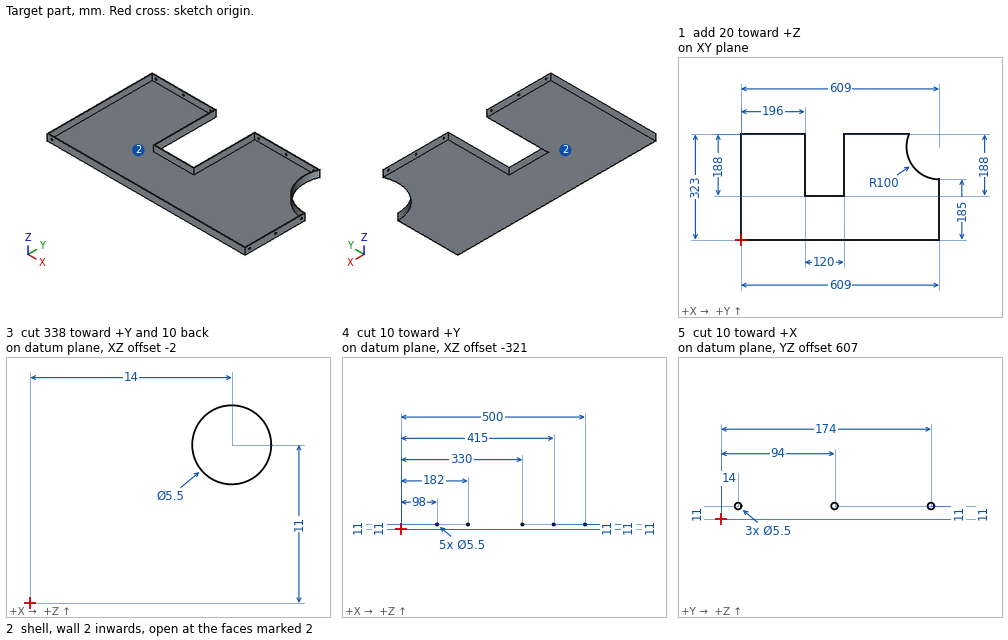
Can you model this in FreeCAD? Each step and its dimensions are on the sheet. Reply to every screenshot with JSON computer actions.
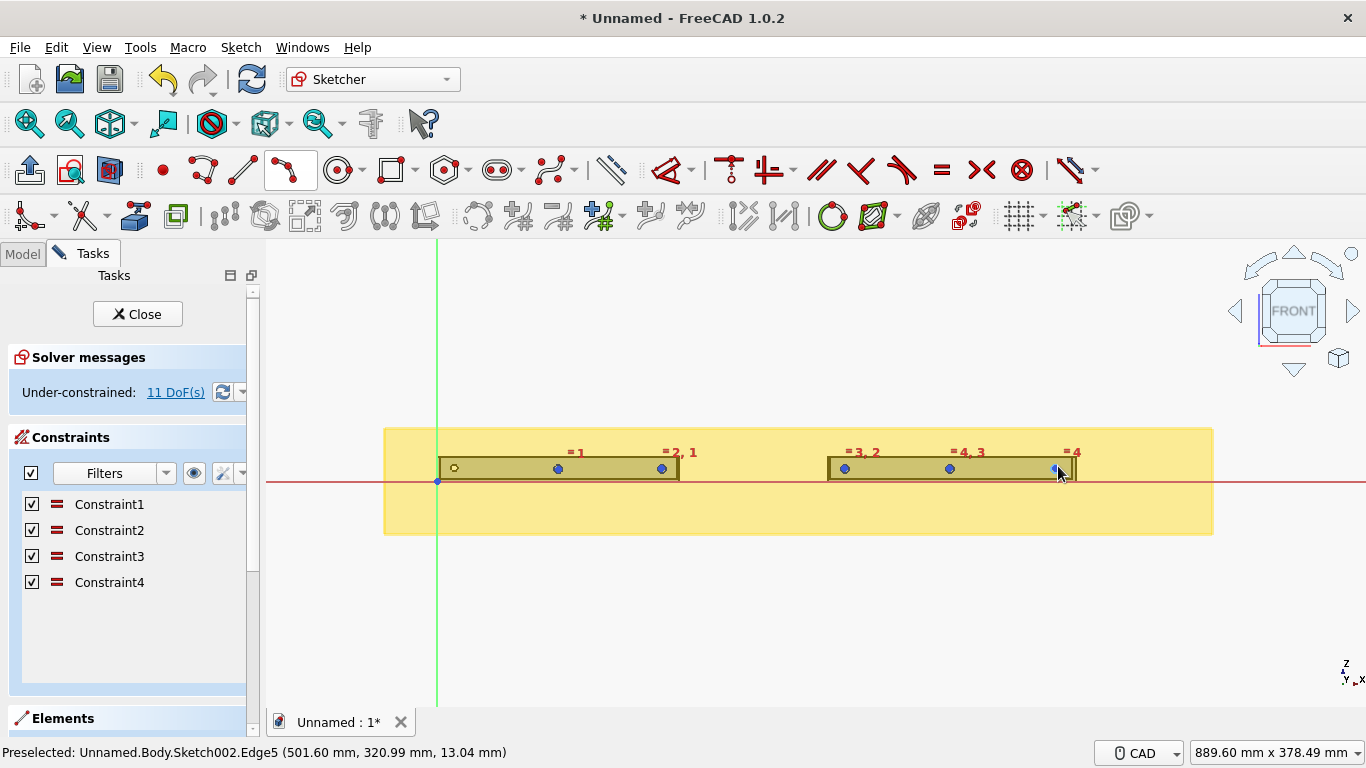
{"action": "scroll", "coordinate": [561, 466], "scroll_direction": "up", "scroll_amount": 9}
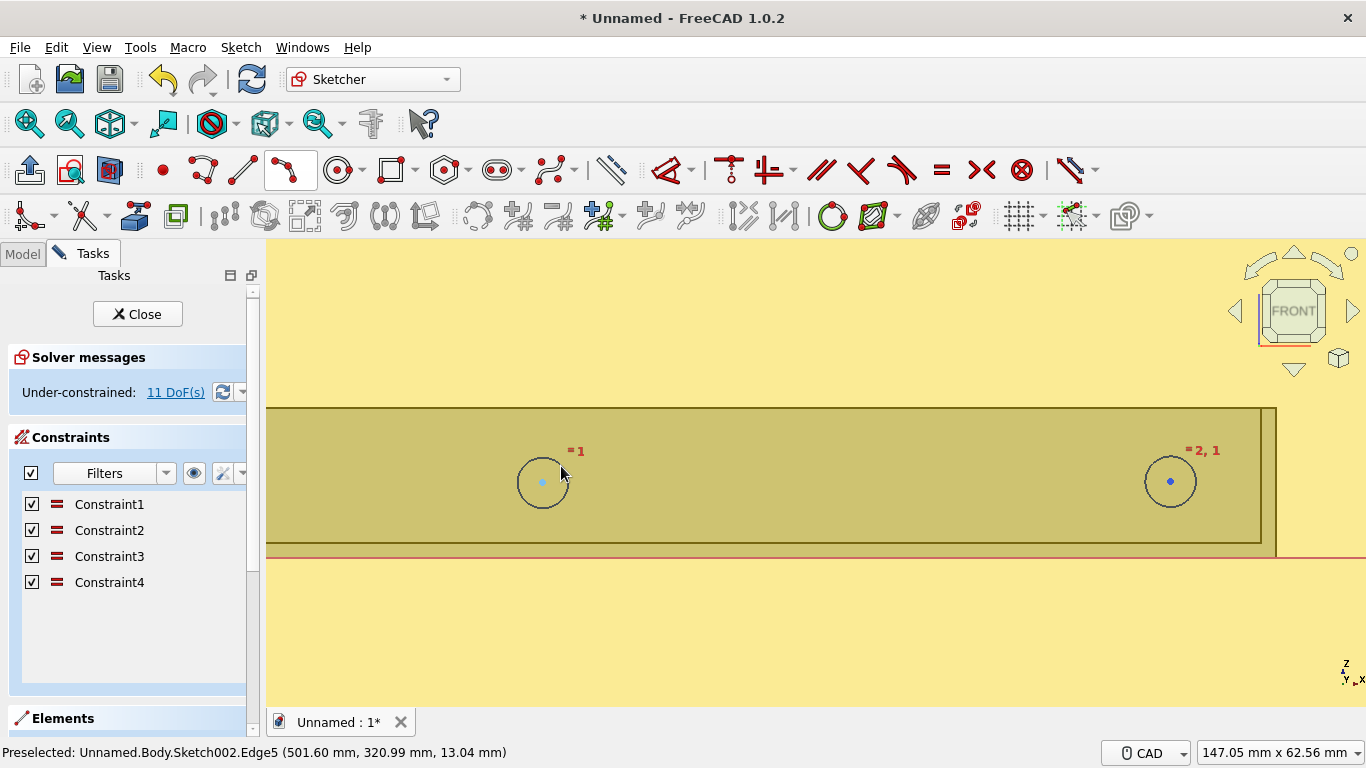
{"action": "left_click", "coordinate": [561, 465]}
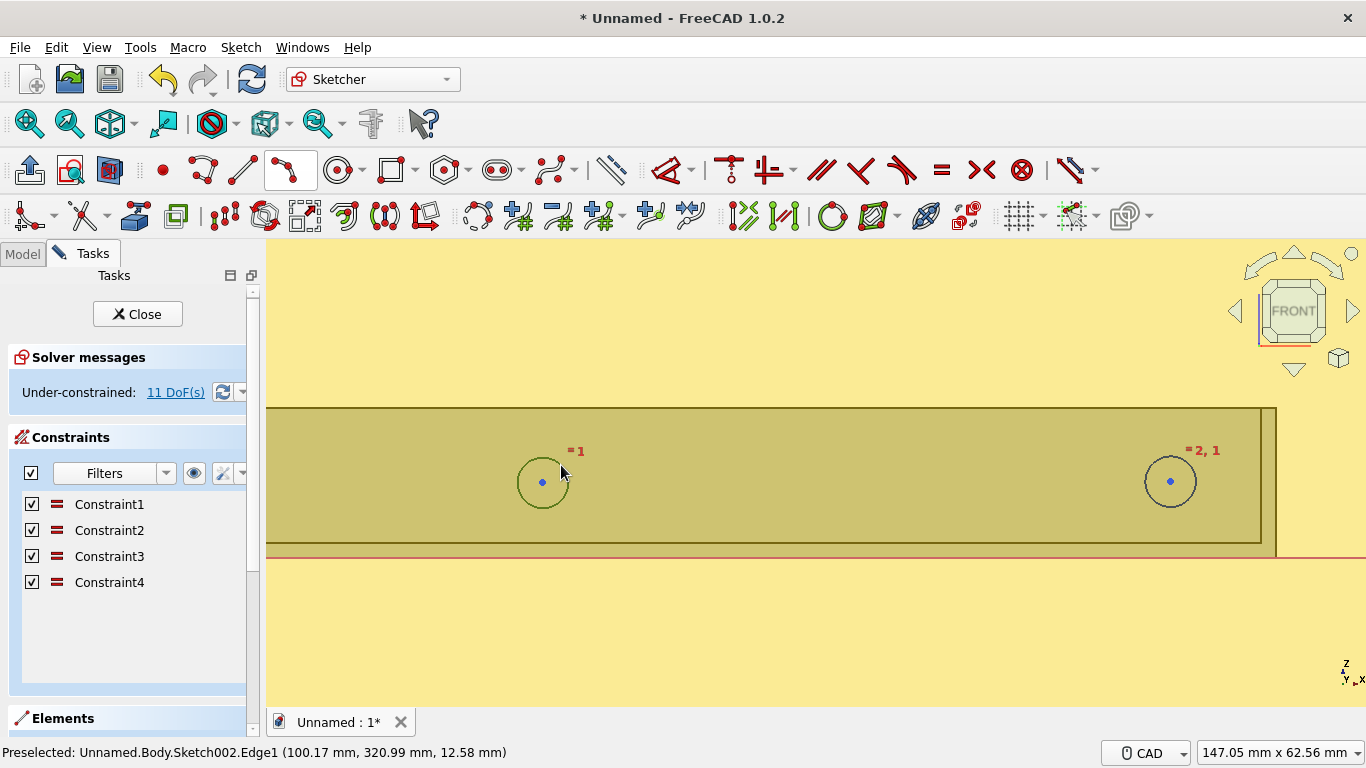
{"action": "key", "text": "k o"}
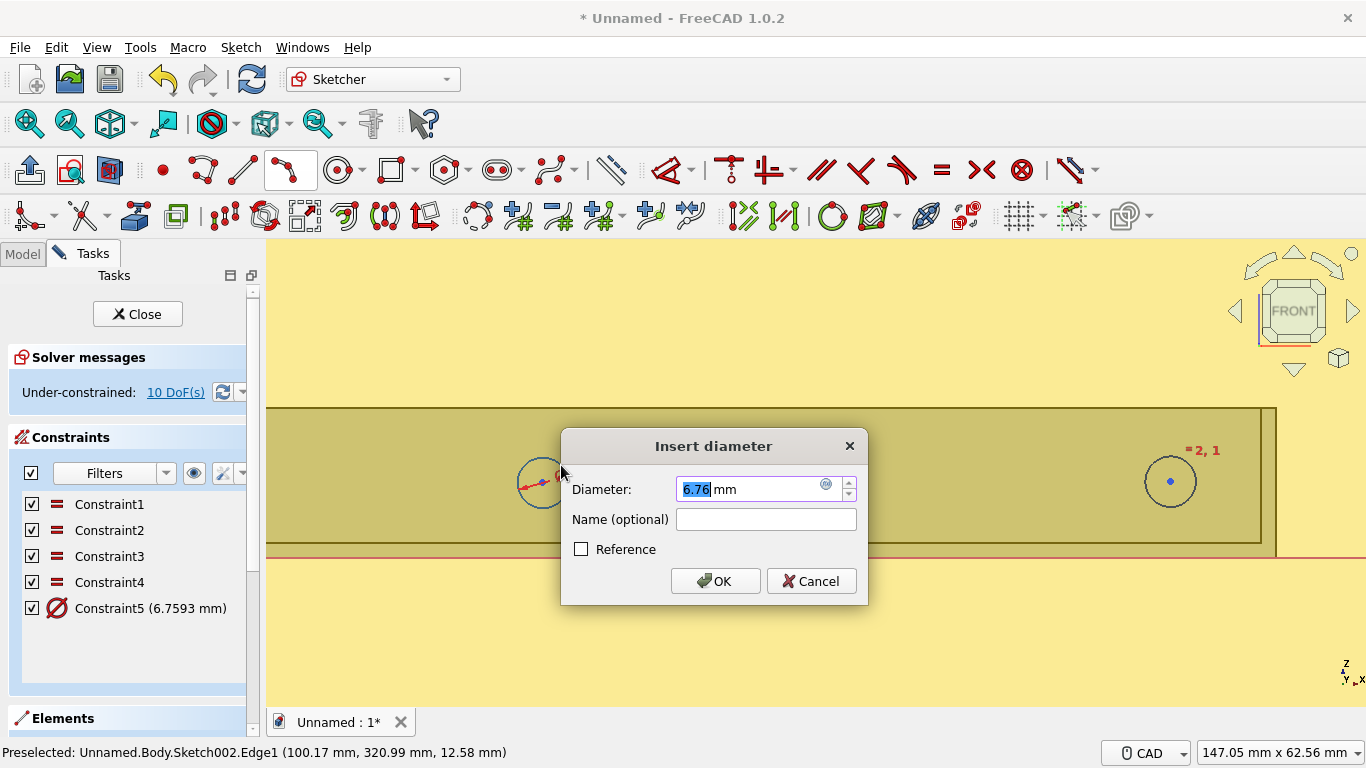
{"action": "type", "text": "5.5"}
{"action": "key", "text": "Return"}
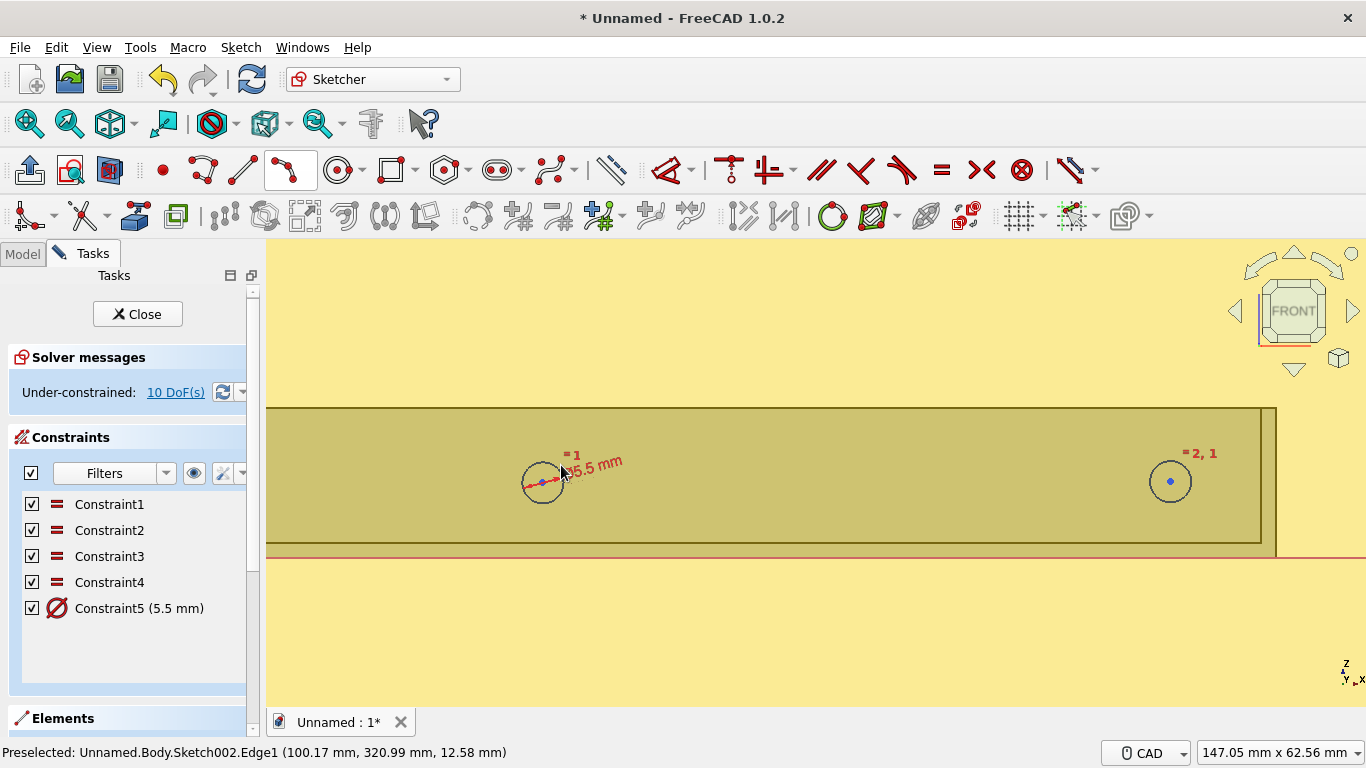
{"action": "scroll", "coordinate": [561, 466], "scroll_direction": "down", "scroll_amount": 9}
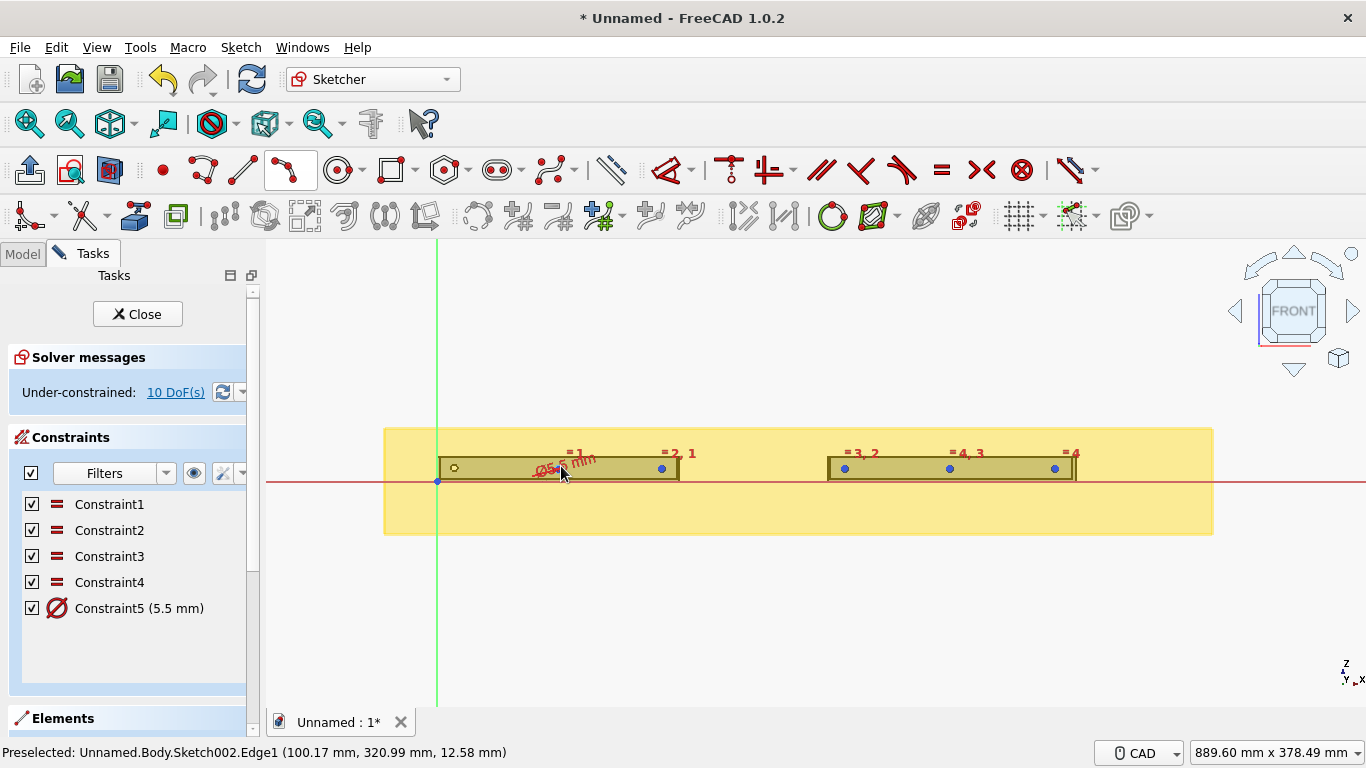
{"action": "left_click", "coordinate": [558, 469]}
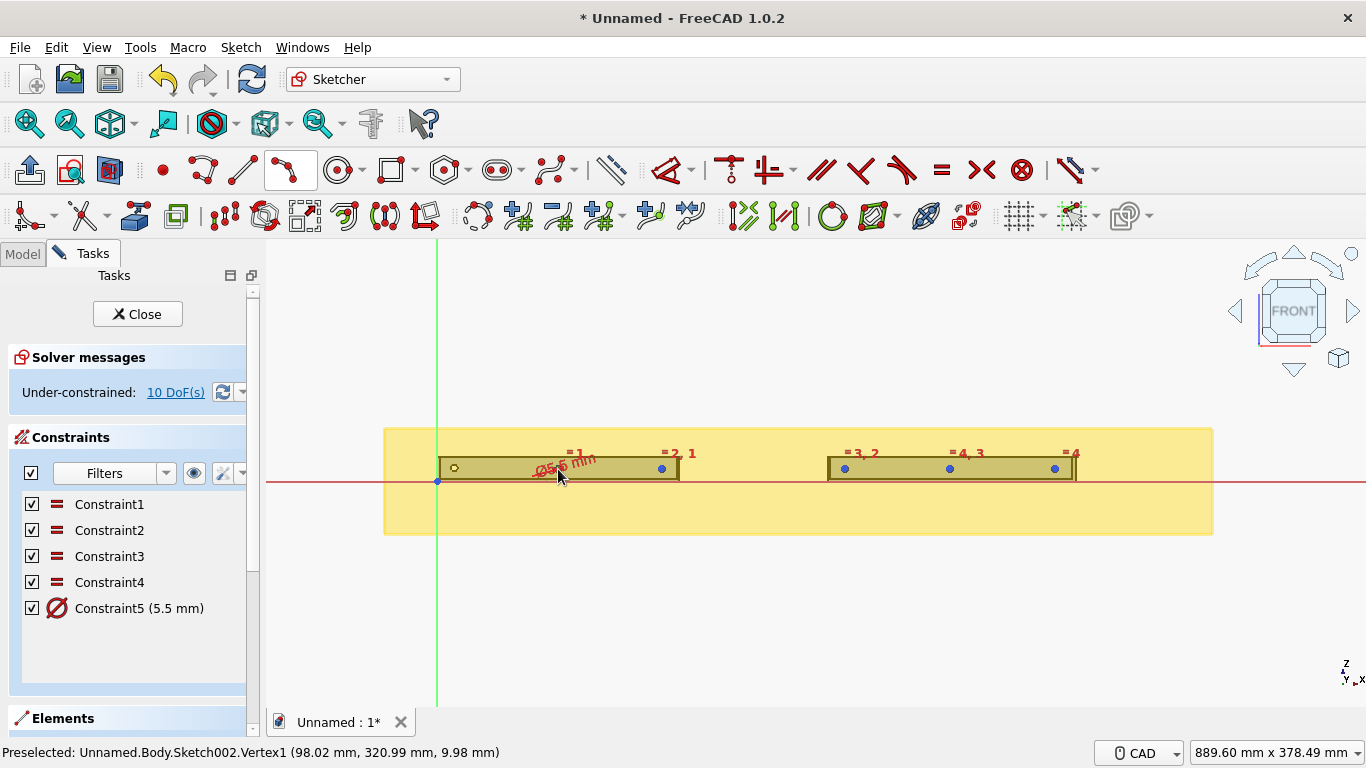
{"action": "key", "text": "l"}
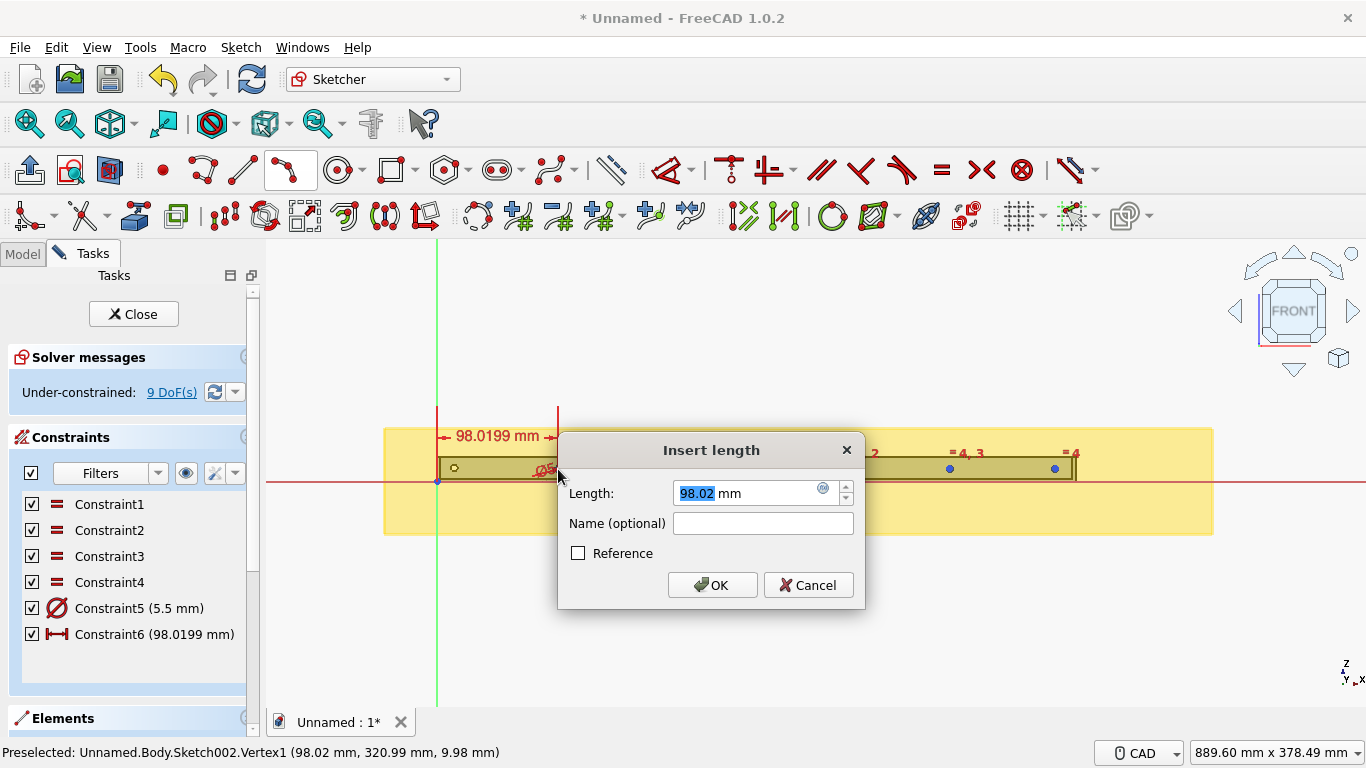
{"action": "type", "text": "98"}
{"action": "key", "text": "Return"}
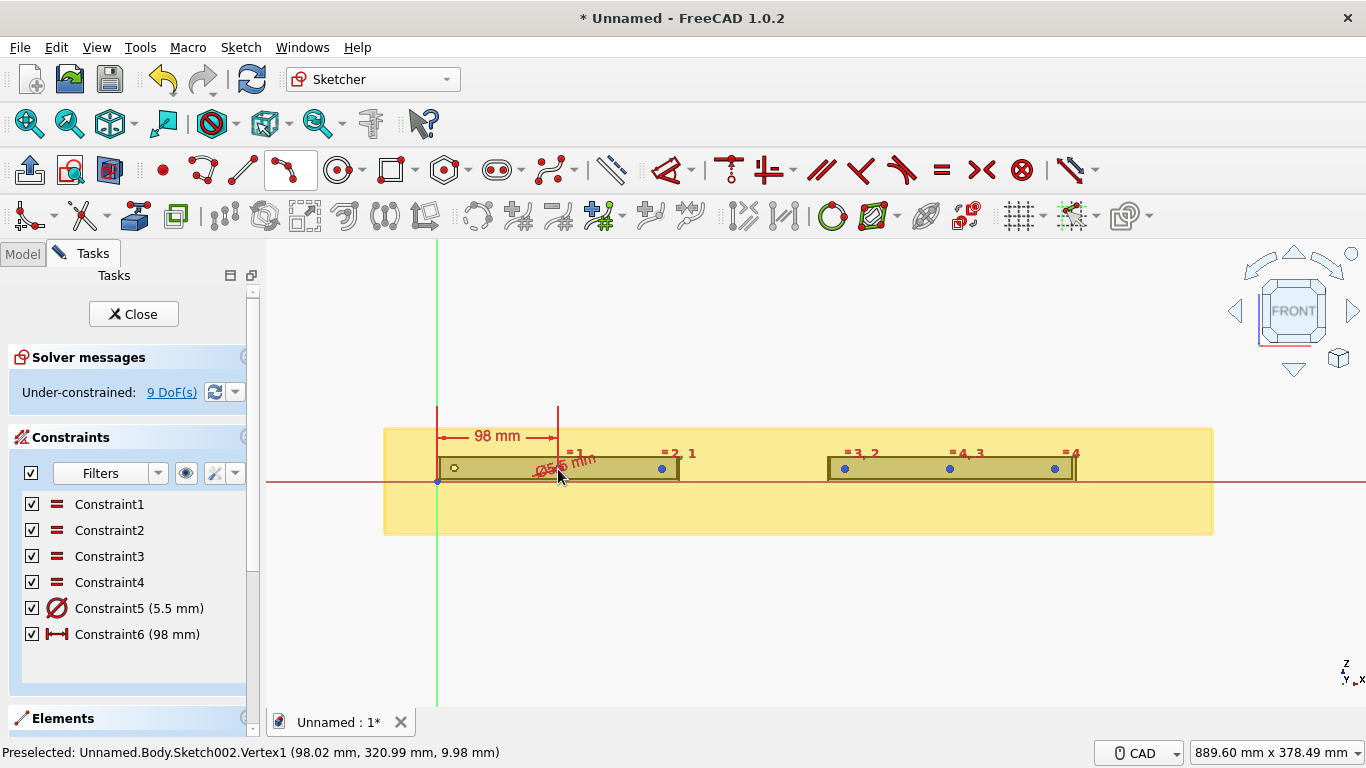
{"action": "scroll", "coordinate": [558, 469], "scroll_direction": "up", "scroll_amount": 6}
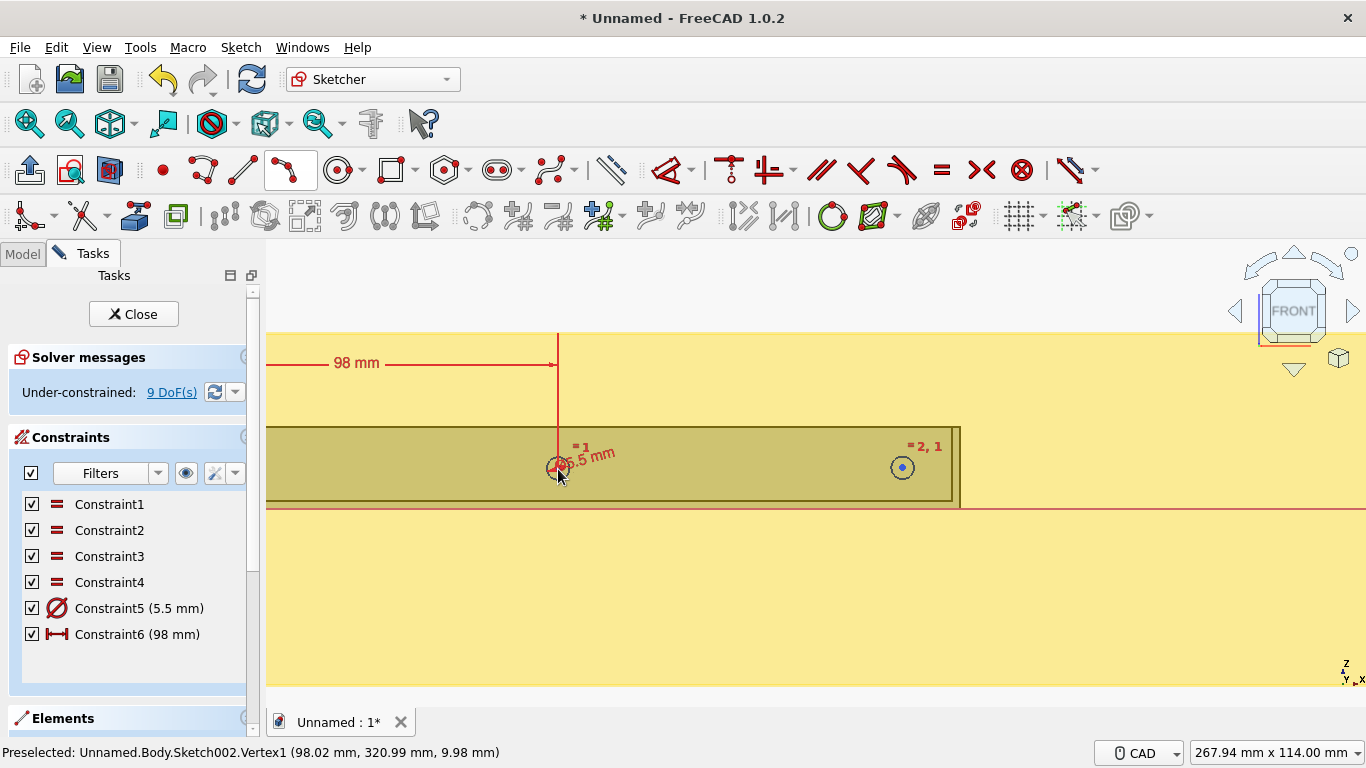
{"action": "left_click", "coordinate": [558, 469]}